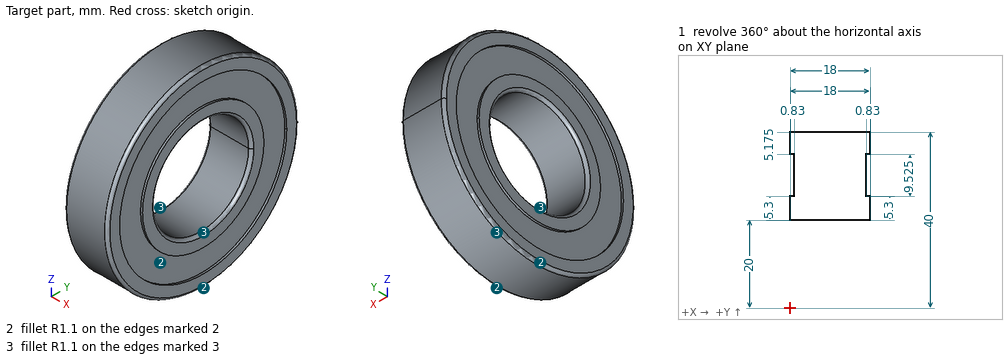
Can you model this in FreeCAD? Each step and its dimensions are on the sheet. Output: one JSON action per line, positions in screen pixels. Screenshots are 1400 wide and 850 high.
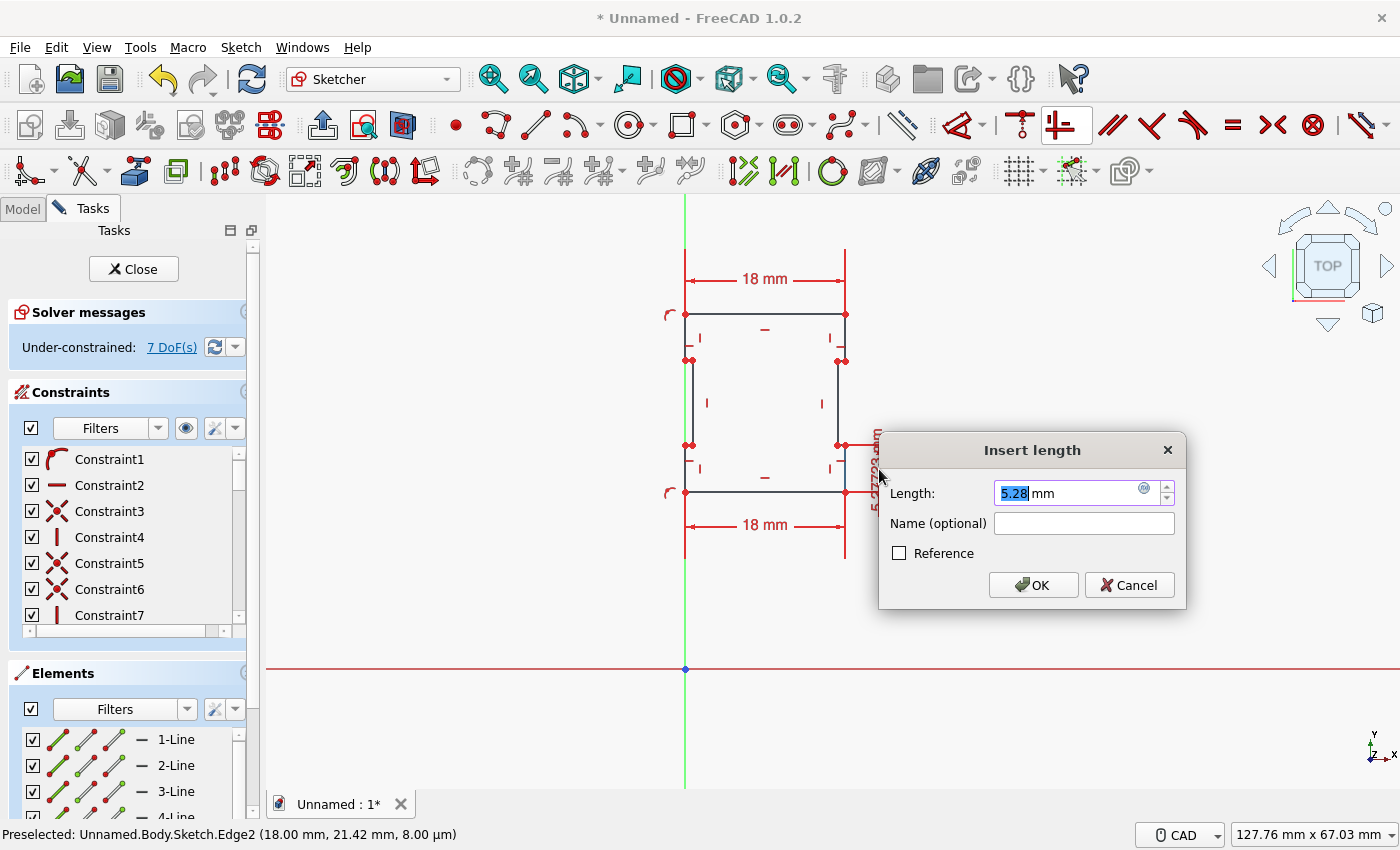
{"action": "type", "text": "5.3"}
{"action": "key", "text": "Return"}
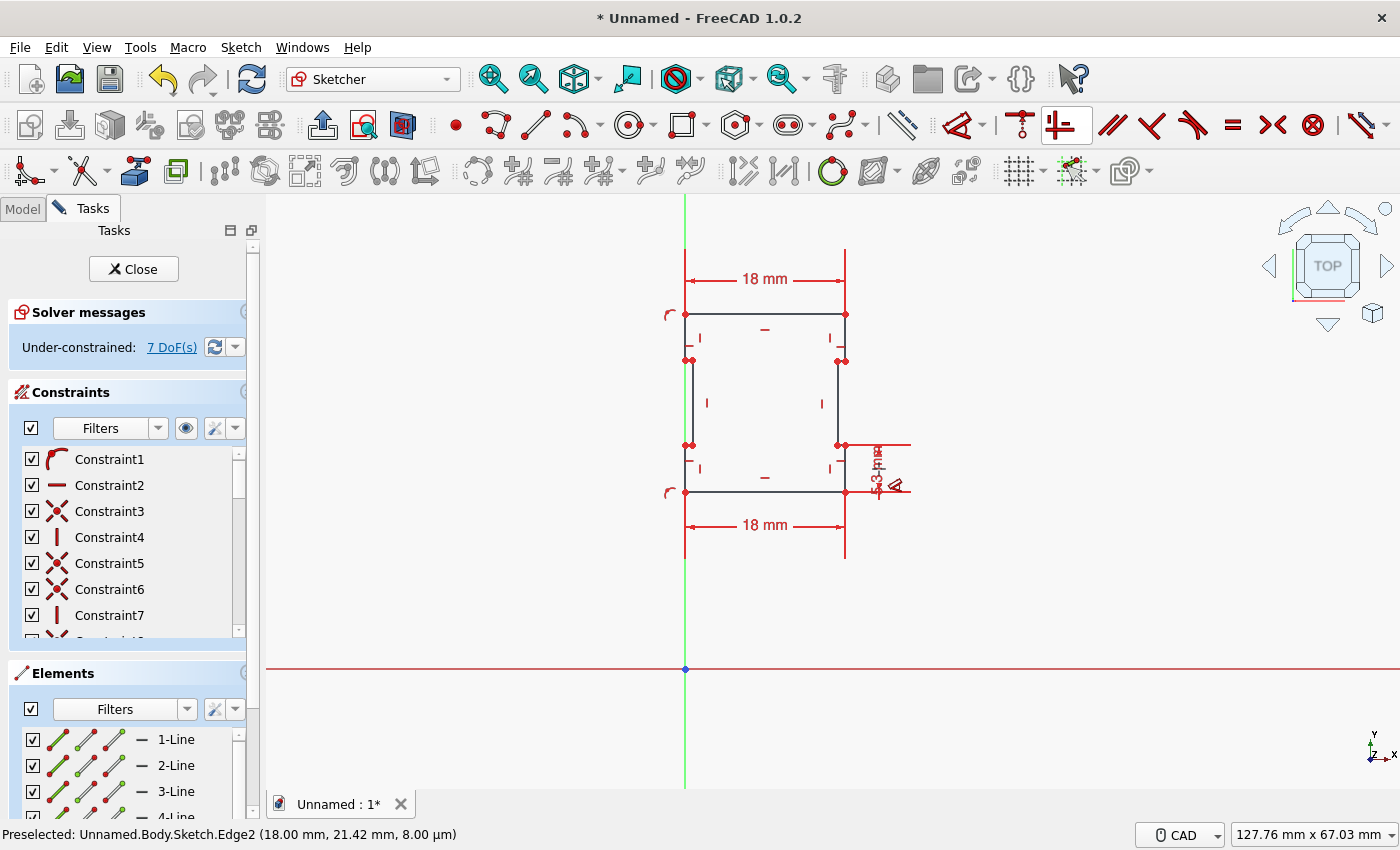
{"action": "left_click", "coordinate": [685, 459]}
{"action": "left_click", "coordinate": [651, 469]}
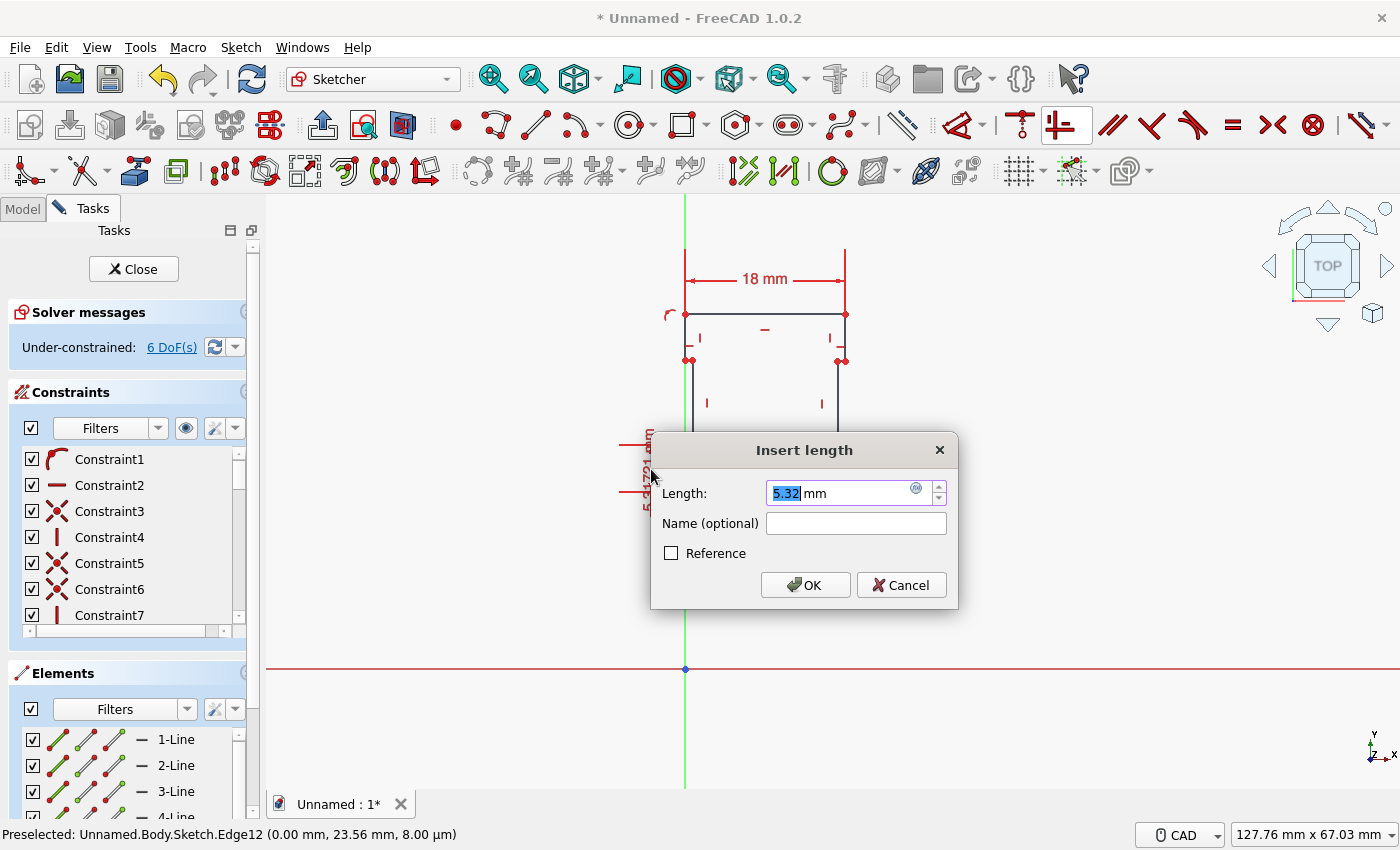
{"action": "type", "text": "5.3"}
{"action": "key", "text": "Return"}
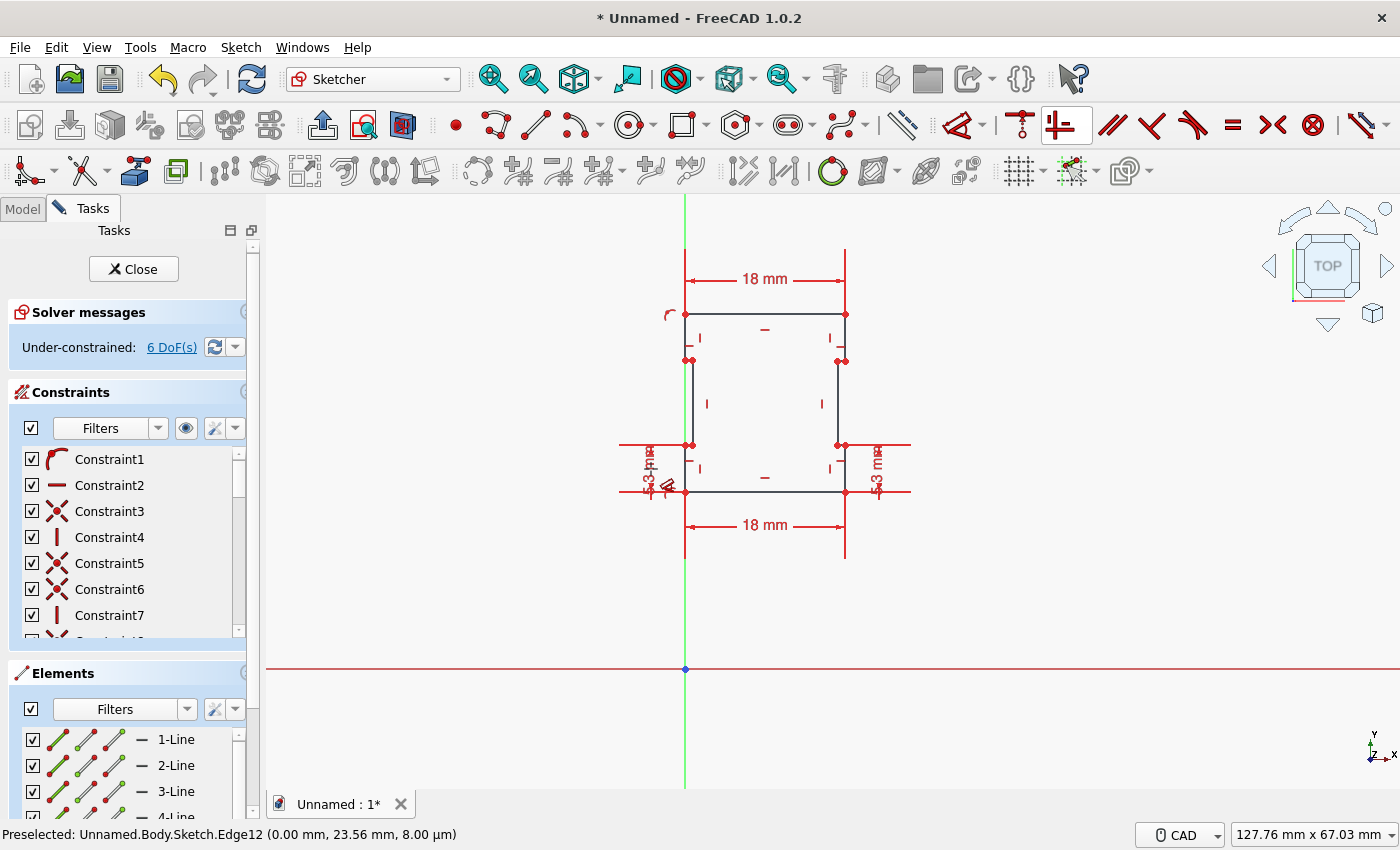
{"action": "left_click", "coordinate": [685, 492]}
{"action": "left_click", "coordinate": [651, 581]}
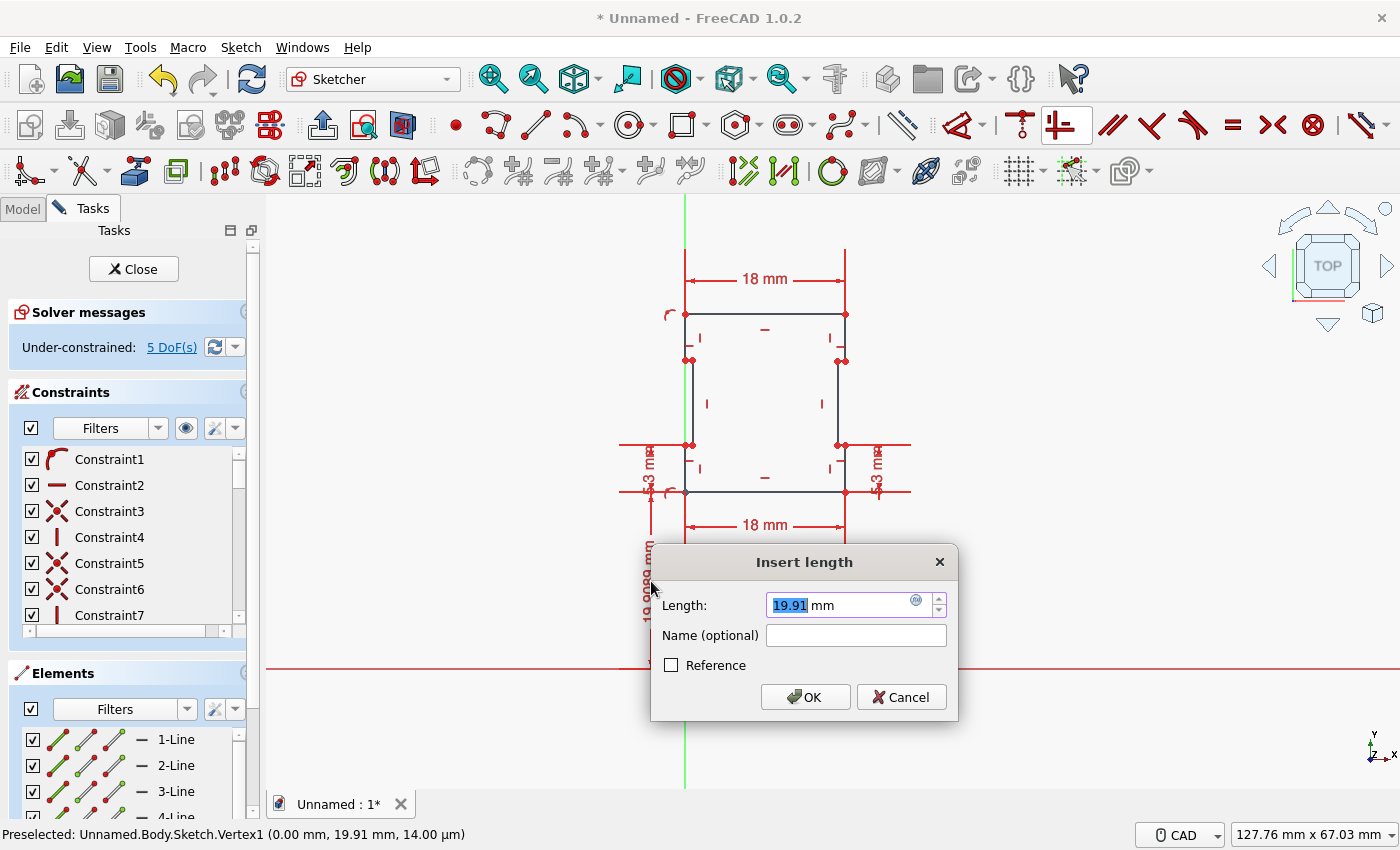
{"action": "type", "text": "20"}
{"action": "key", "text": "Return"}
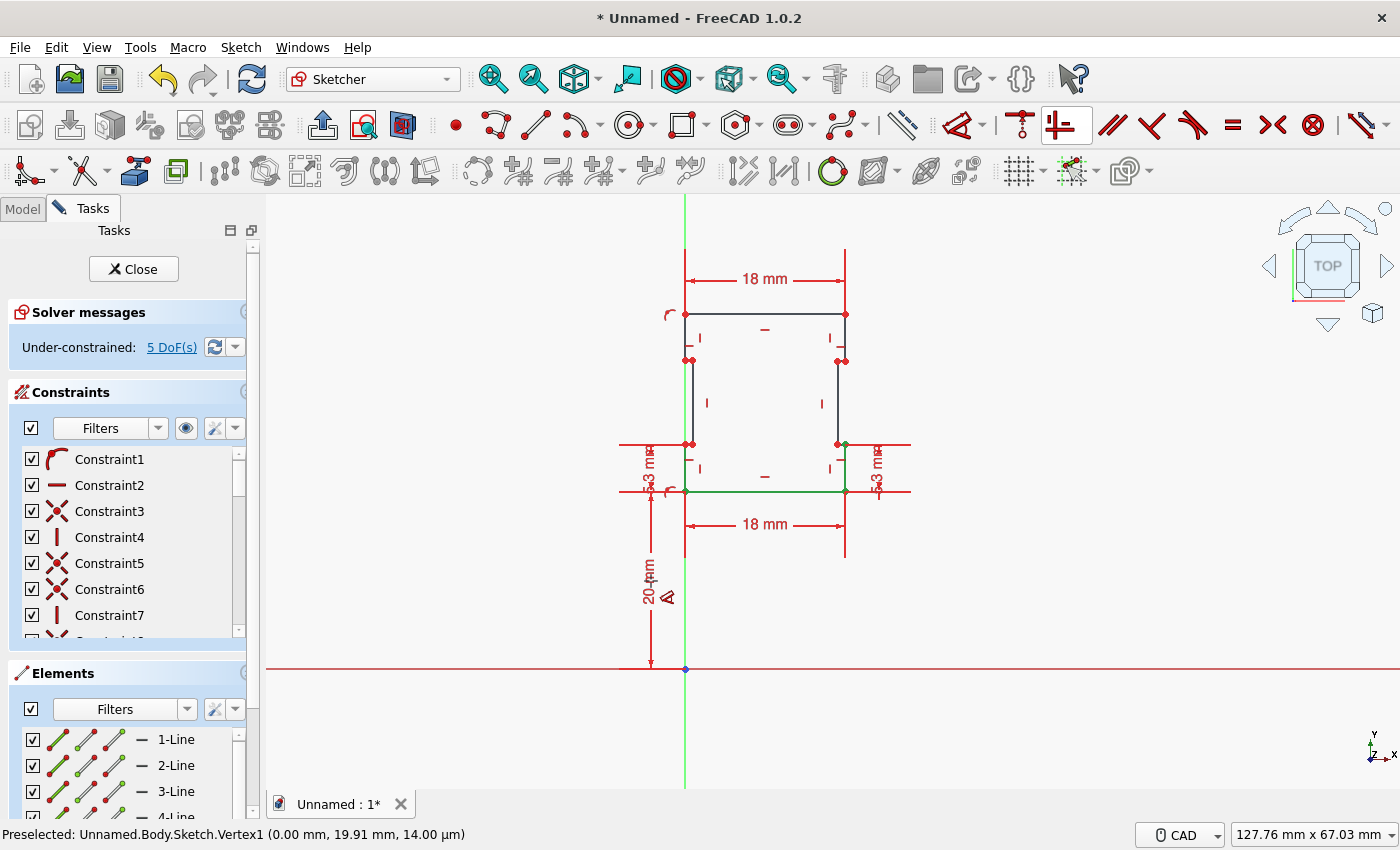
{"action": "left_click", "coordinate": [845, 314]}
{"action": "left_click", "coordinate": [879, 492]}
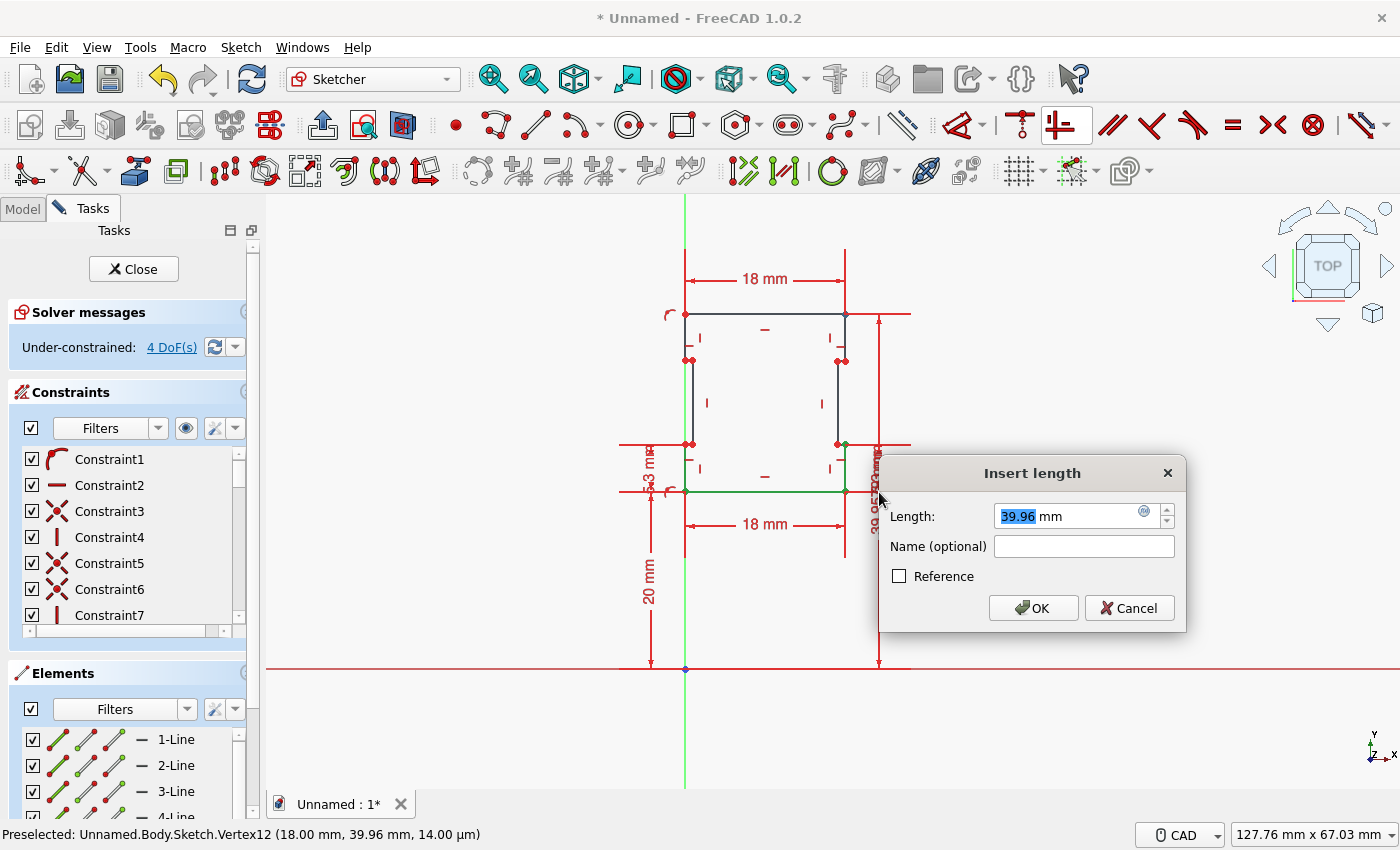
{"action": "type", "text": "40"}
{"action": "key", "text": "Return"}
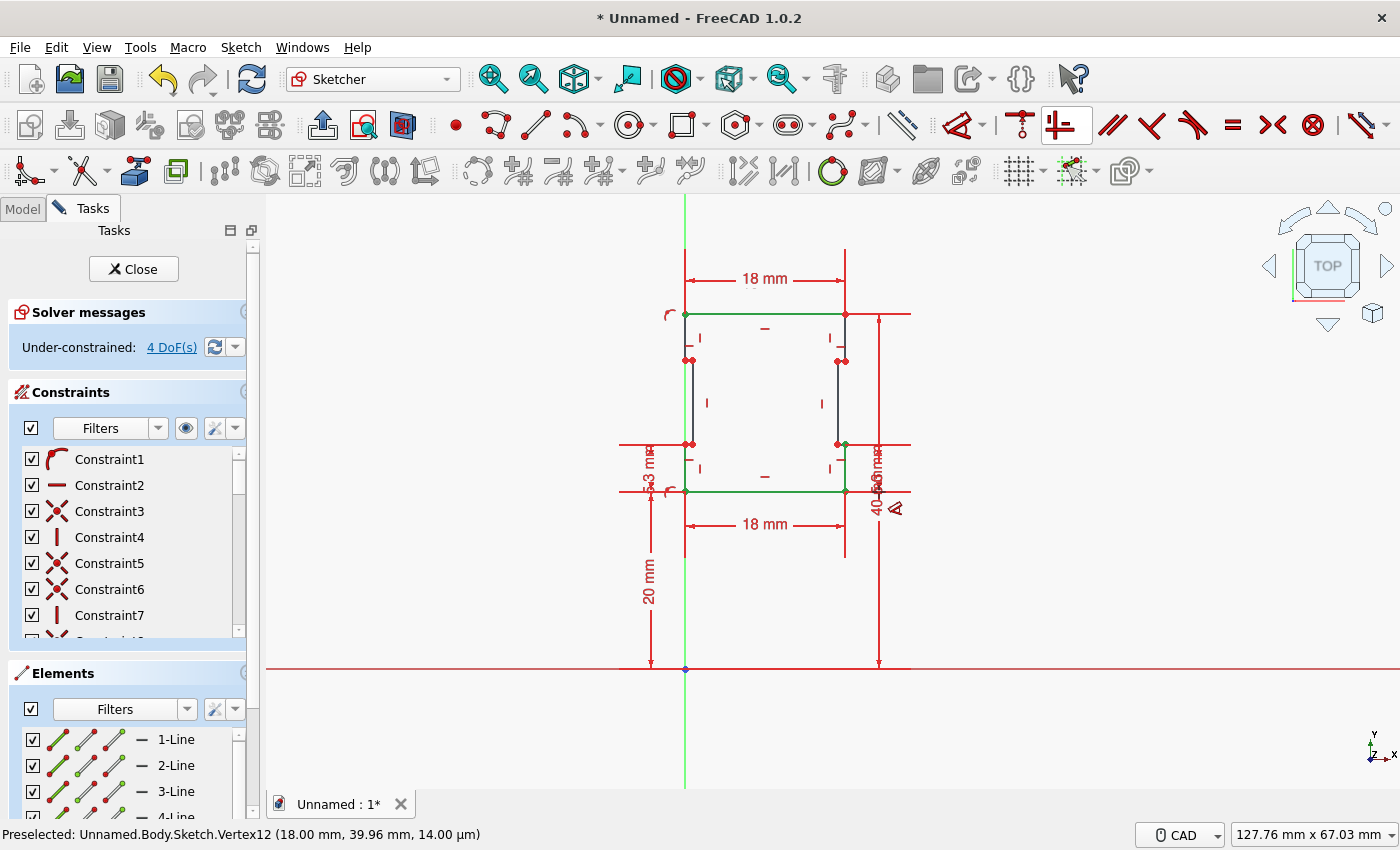
{"action": "scroll", "coordinate": [841, 445], "scroll_direction": "up", "scroll_amount": 9}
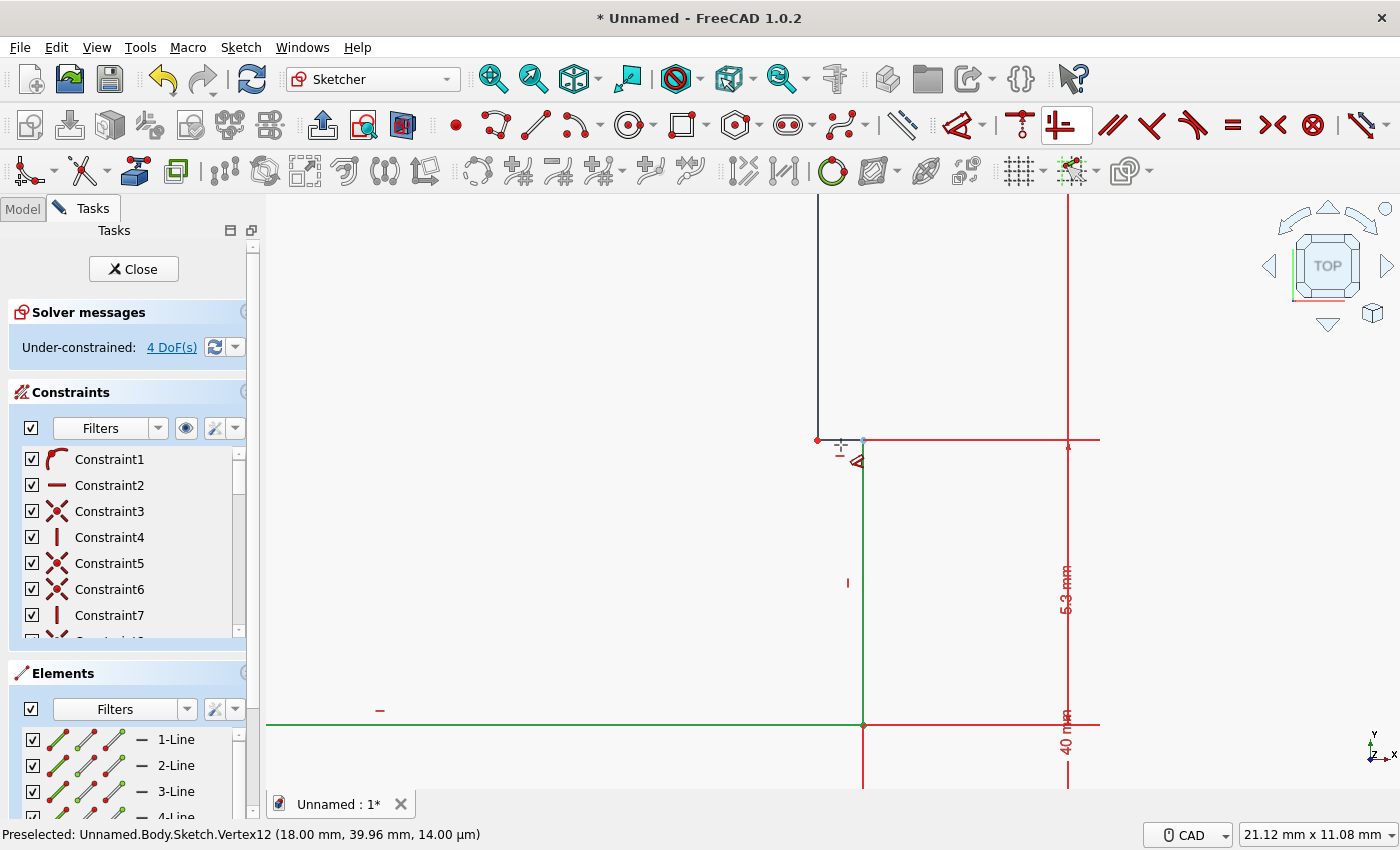
{"action": "left_click", "coordinate": [840, 440]}
{"action": "left_click", "coordinate": [840, 406]}